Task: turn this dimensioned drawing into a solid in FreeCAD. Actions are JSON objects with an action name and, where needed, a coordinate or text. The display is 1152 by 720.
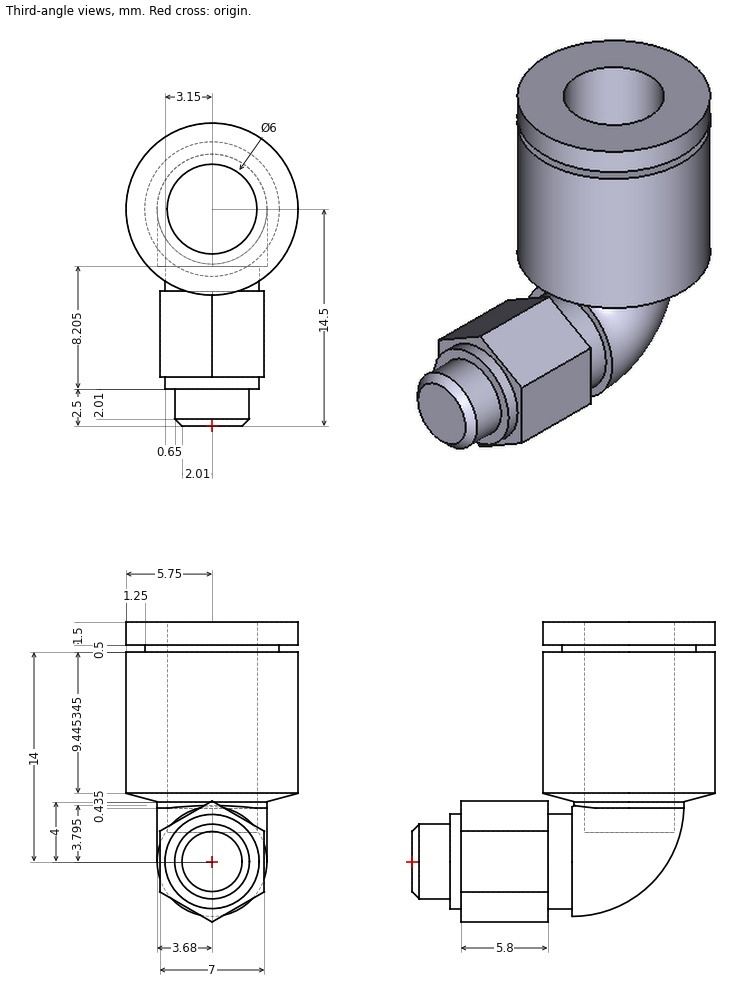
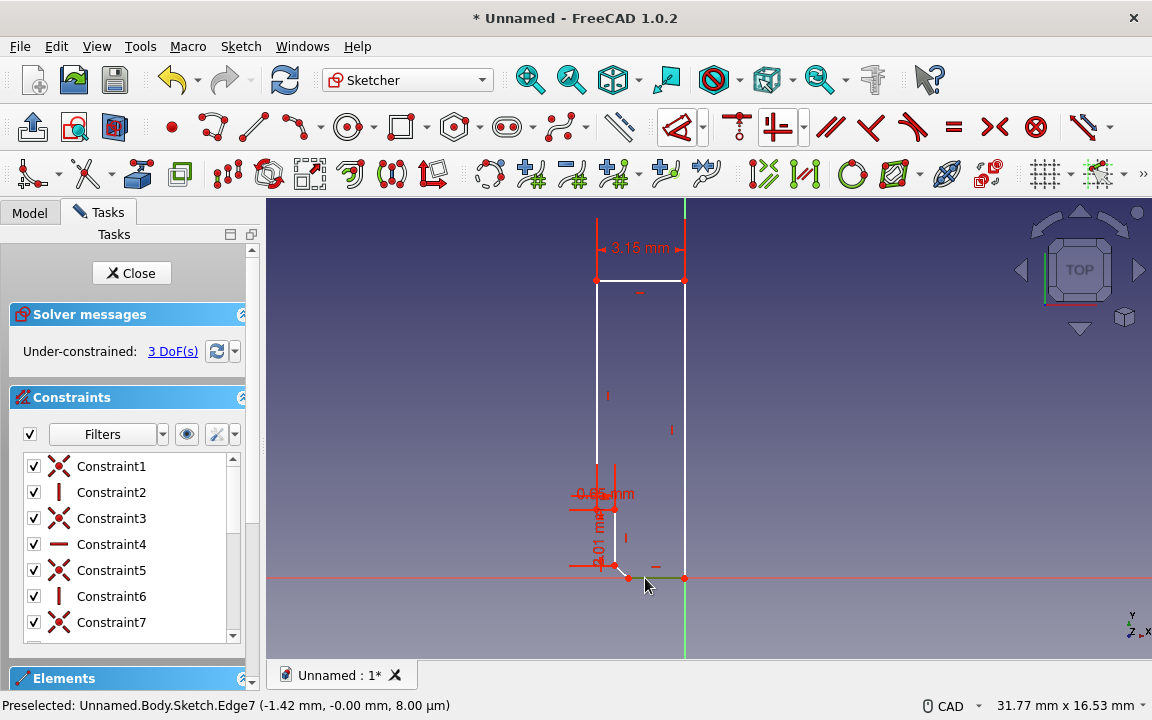
{"action": "left_click", "coordinate": [702, 128]}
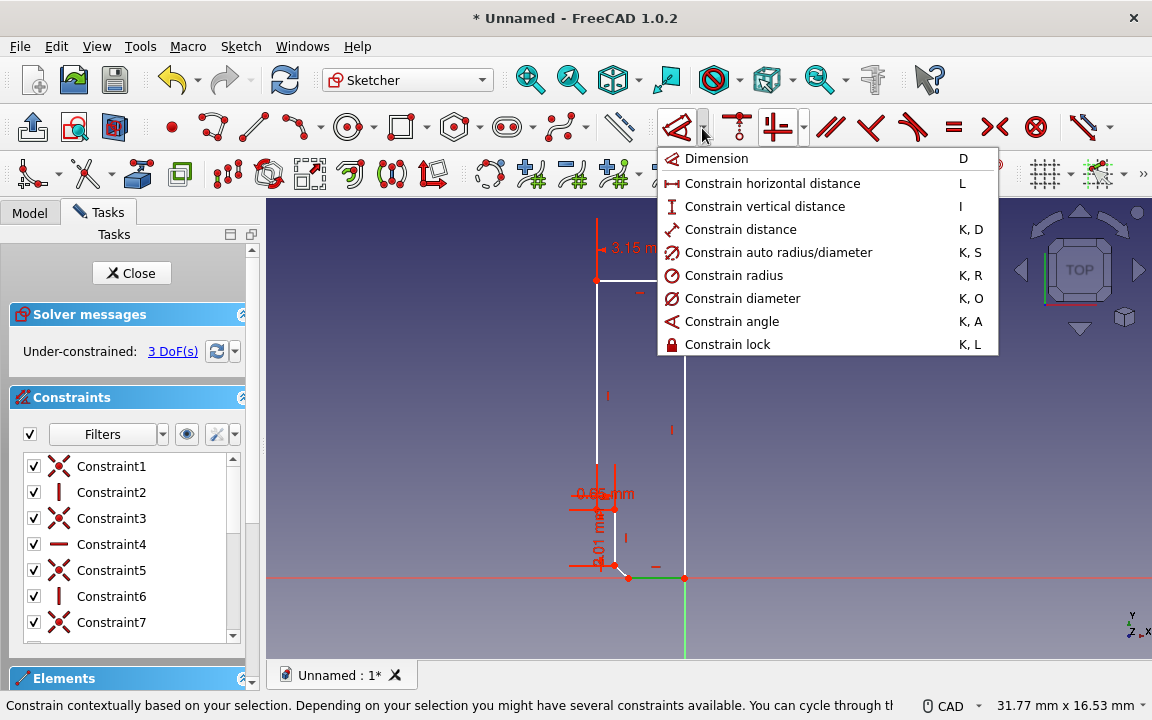
{"action": "left_click", "coordinate": [828, 184]}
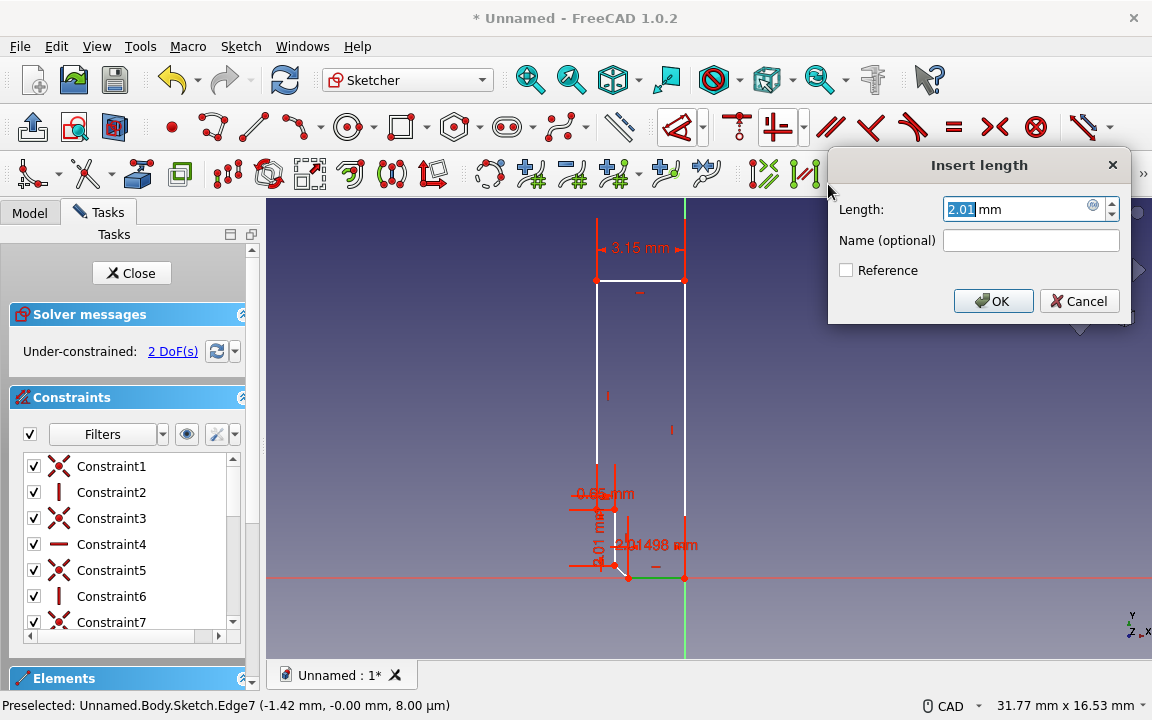
{"action": "type", "text": "2.01"}
{"action": "key", "text": "Return"}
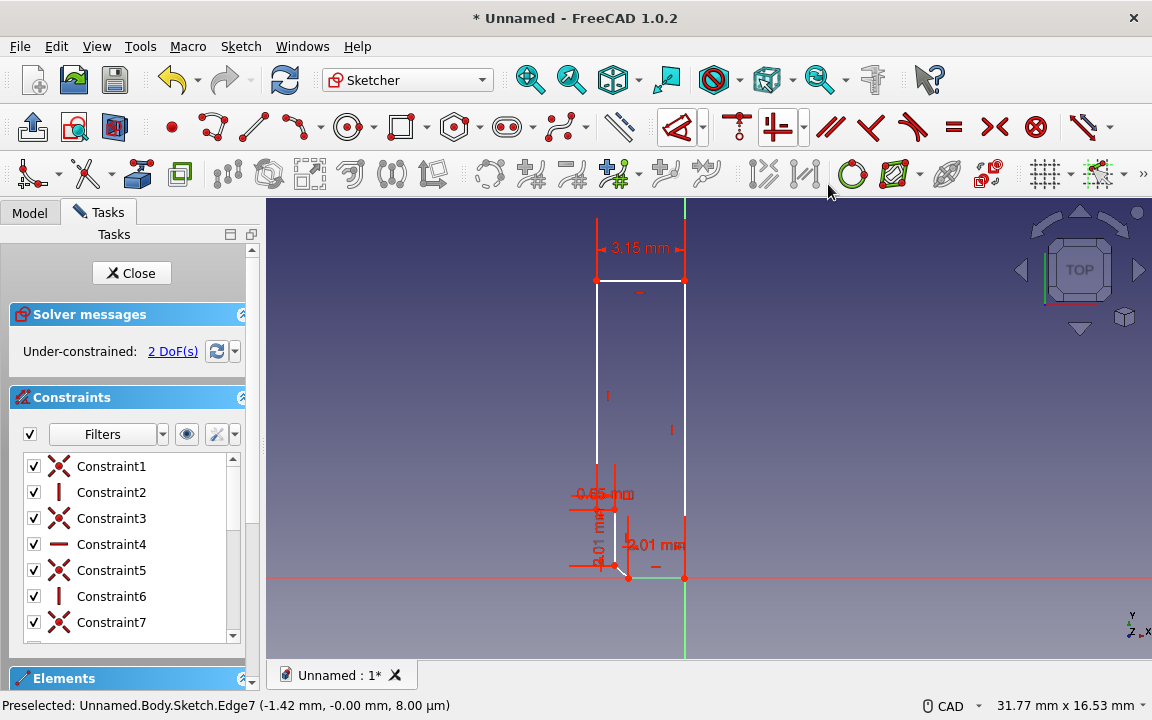
{"action": "left_click", "coordinate": [597, 510]}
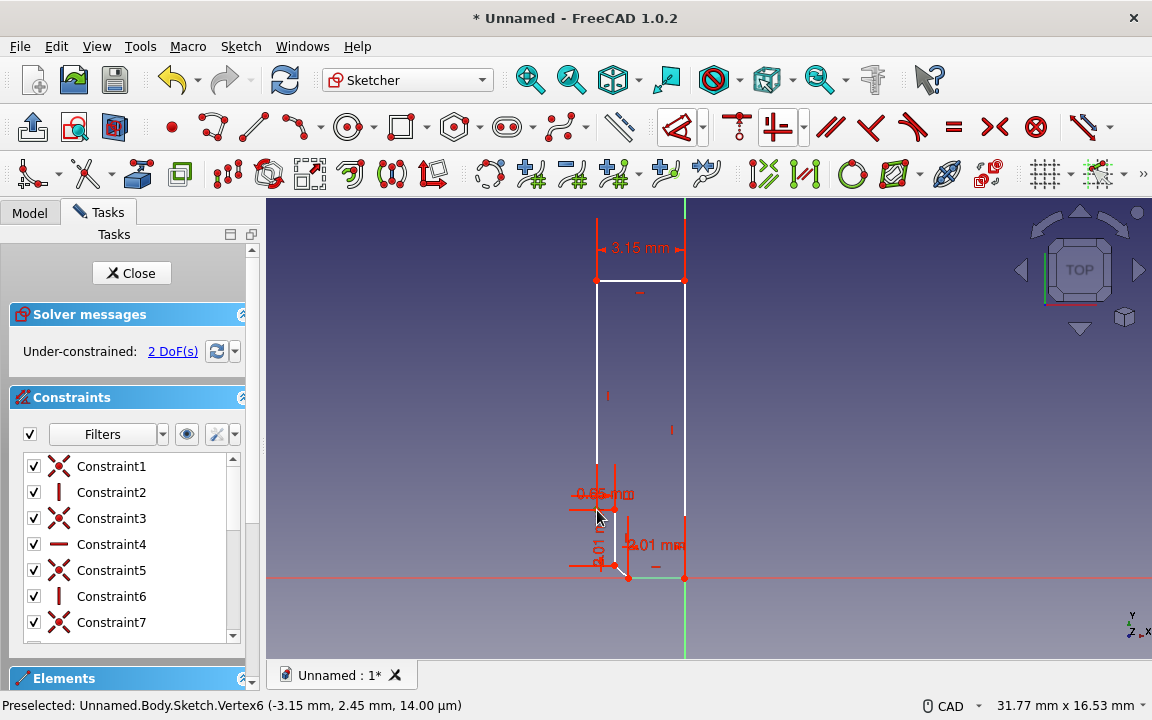
{"action": "key", "text": "i"}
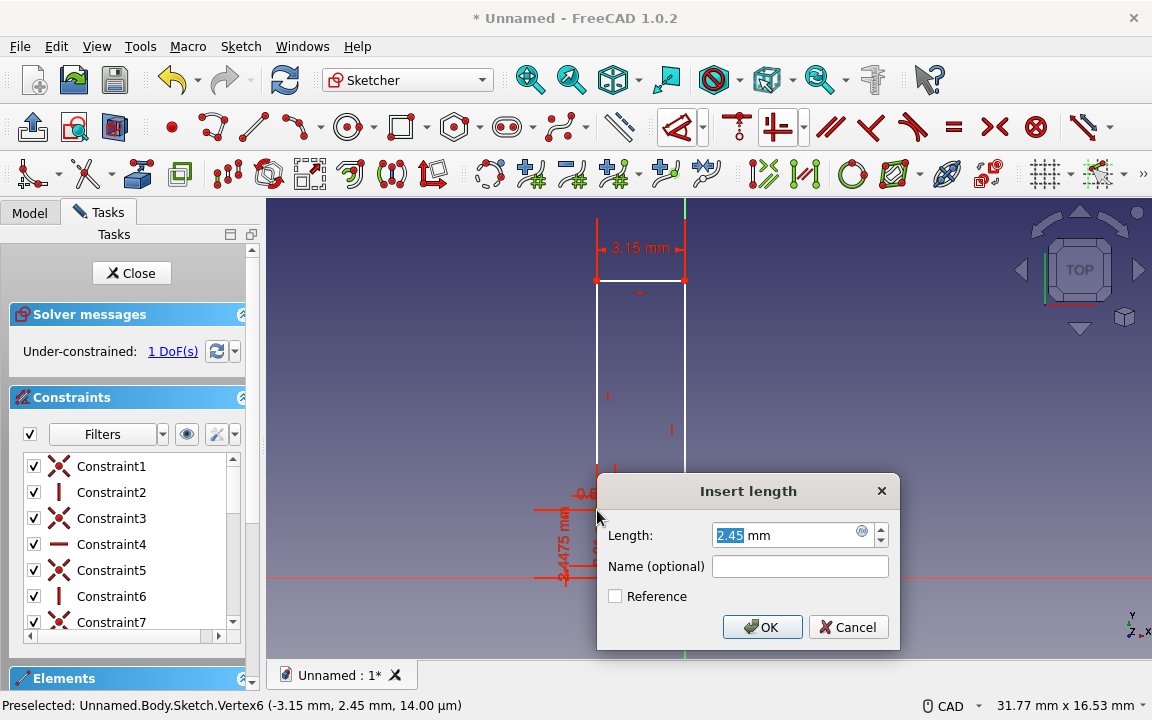
{"action": "type", "text": "2.5"}
{"action": "key", "text": "Return"}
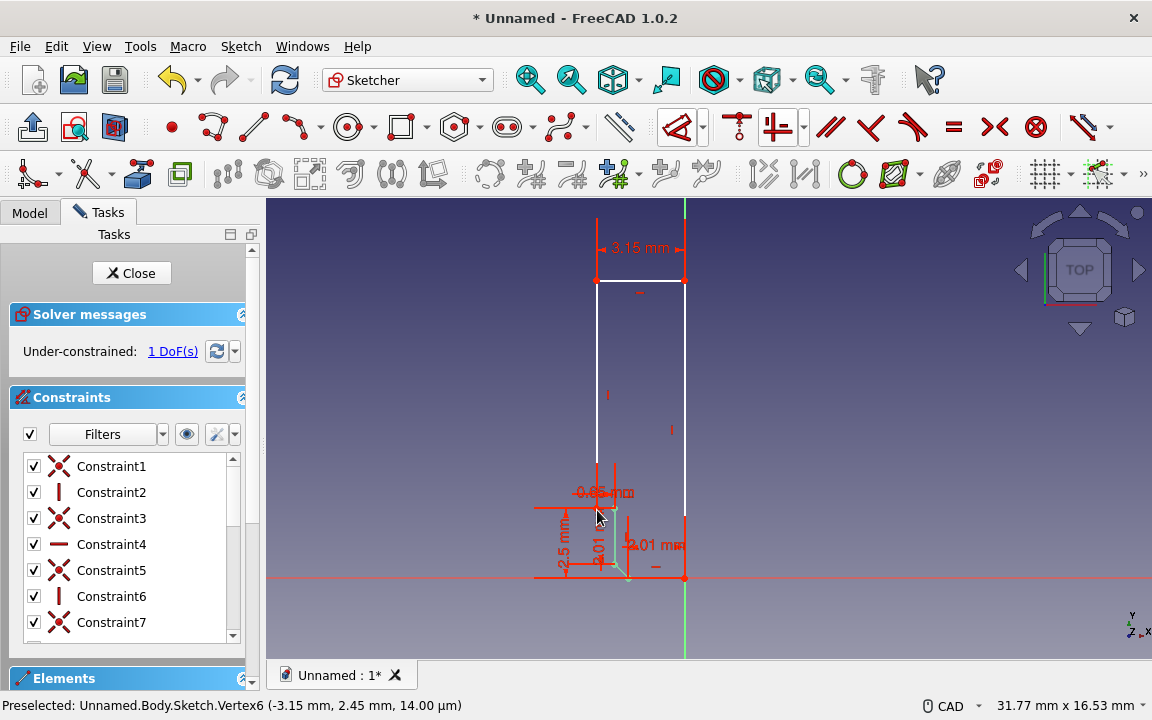
{"action": "left_click", "coordinate": [597, 349]}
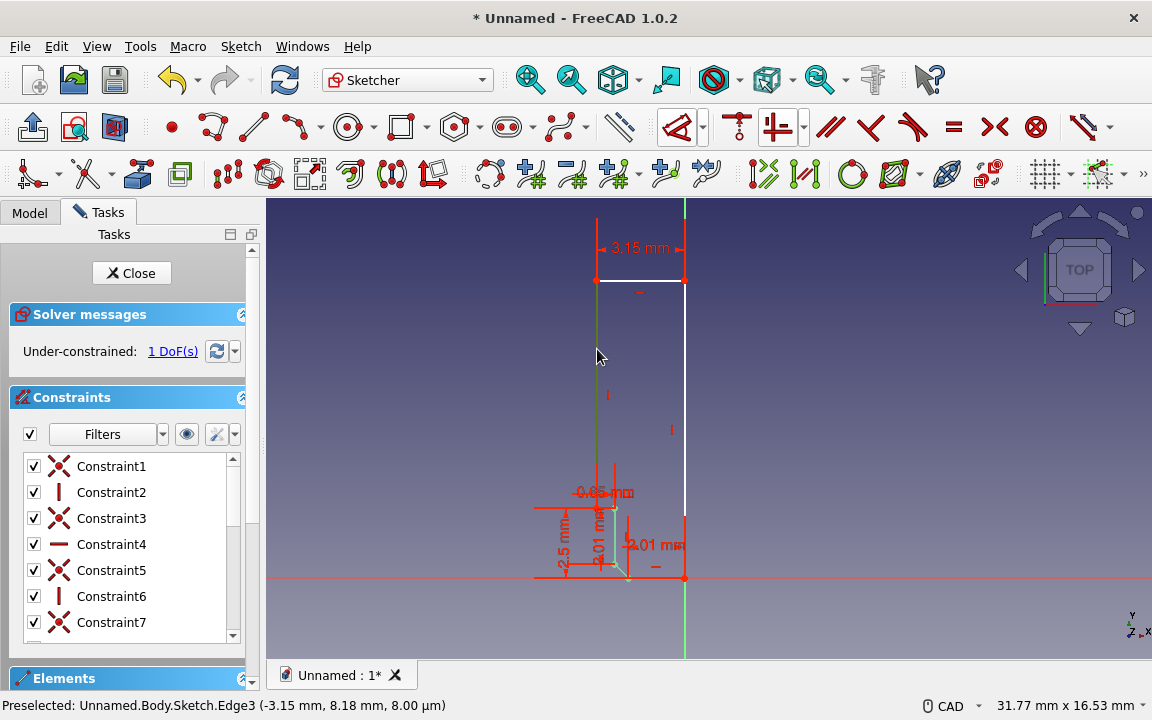
{"action": "key", "text": "i"}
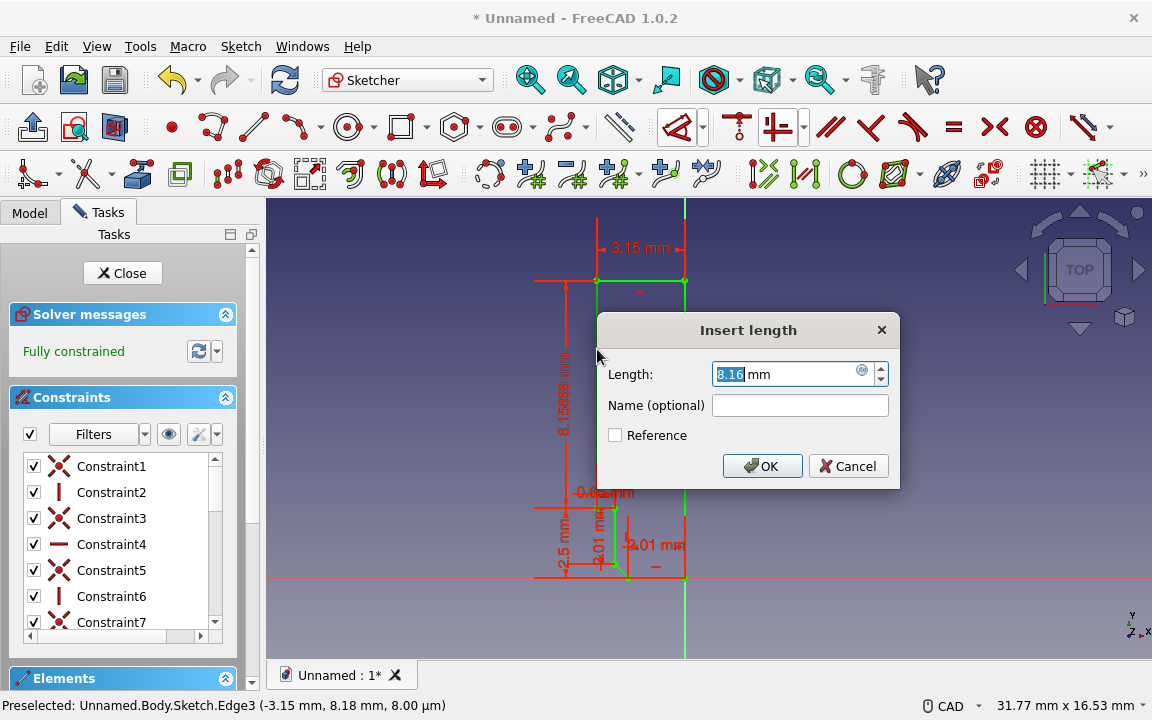
{"action": "type", "text": "8.205"}
{"action": "key", "text": "Return"}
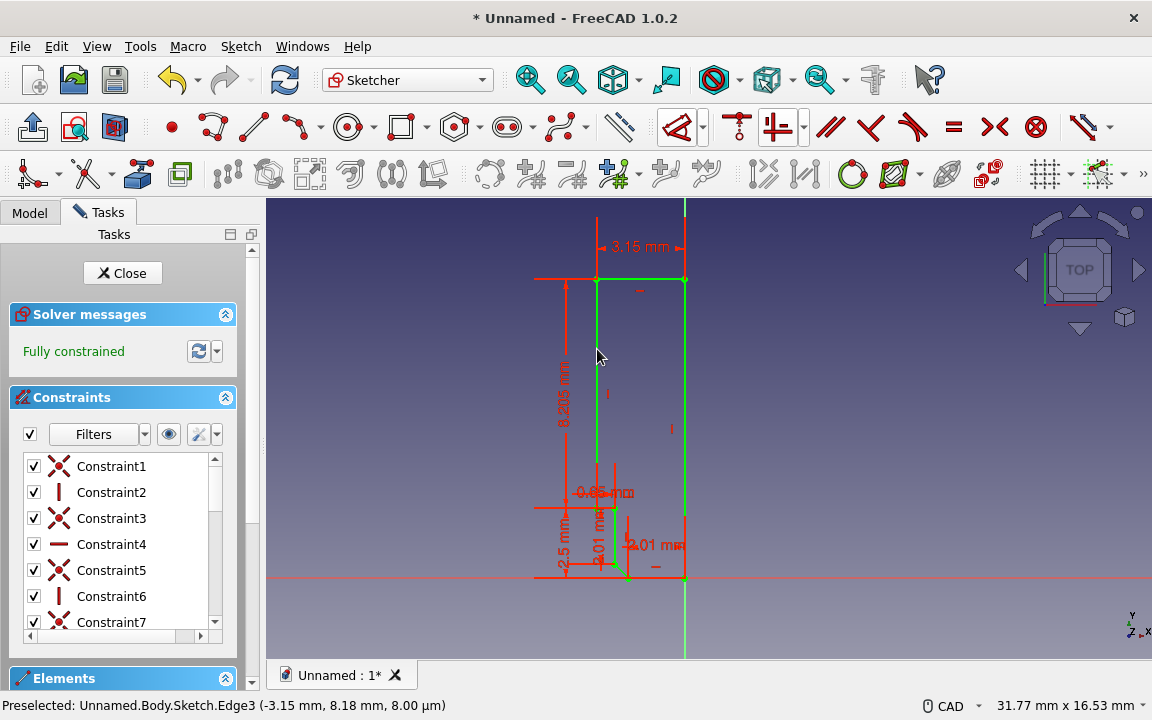
{"action": "left_click", "coordinate": [123, 273]}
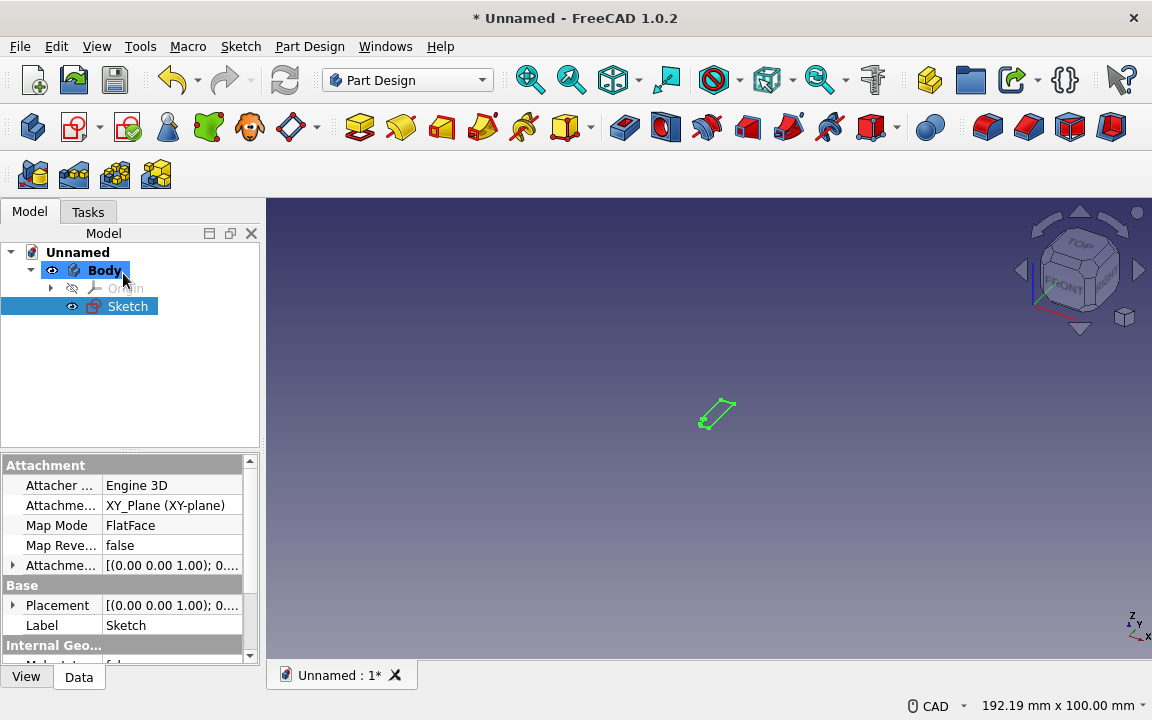
{"action": "left_click", "coordinate": [401, 128]}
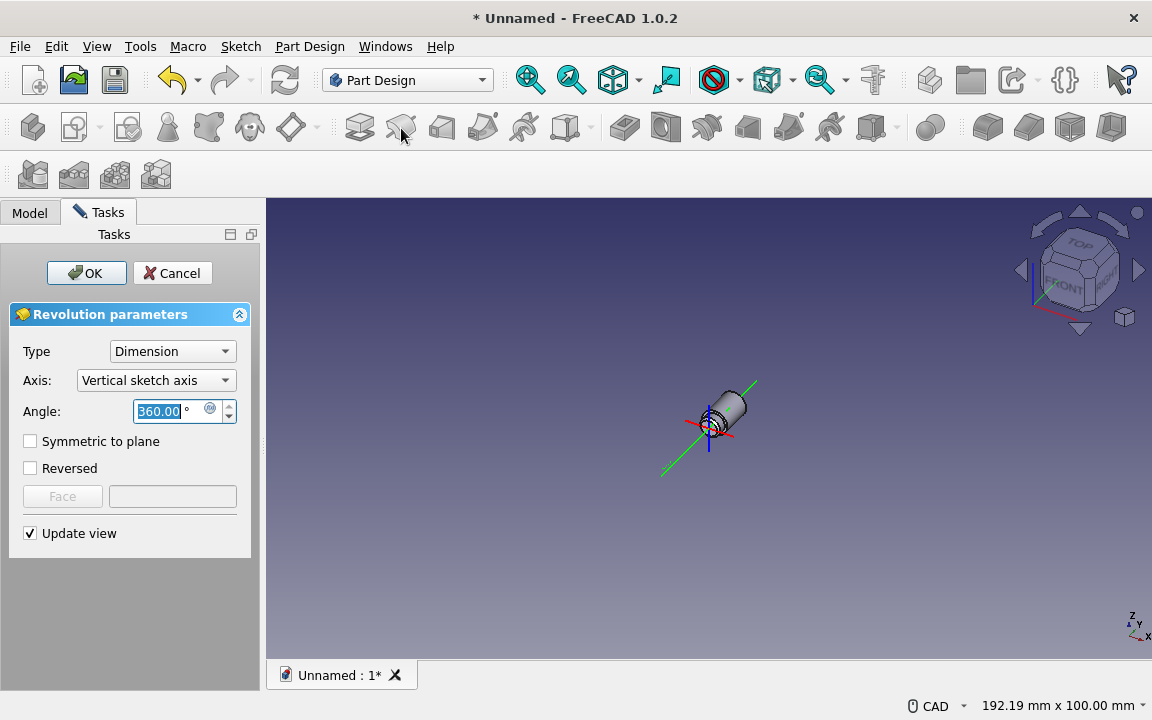
{"action": "left_click", "coordinate": [87, 273]}